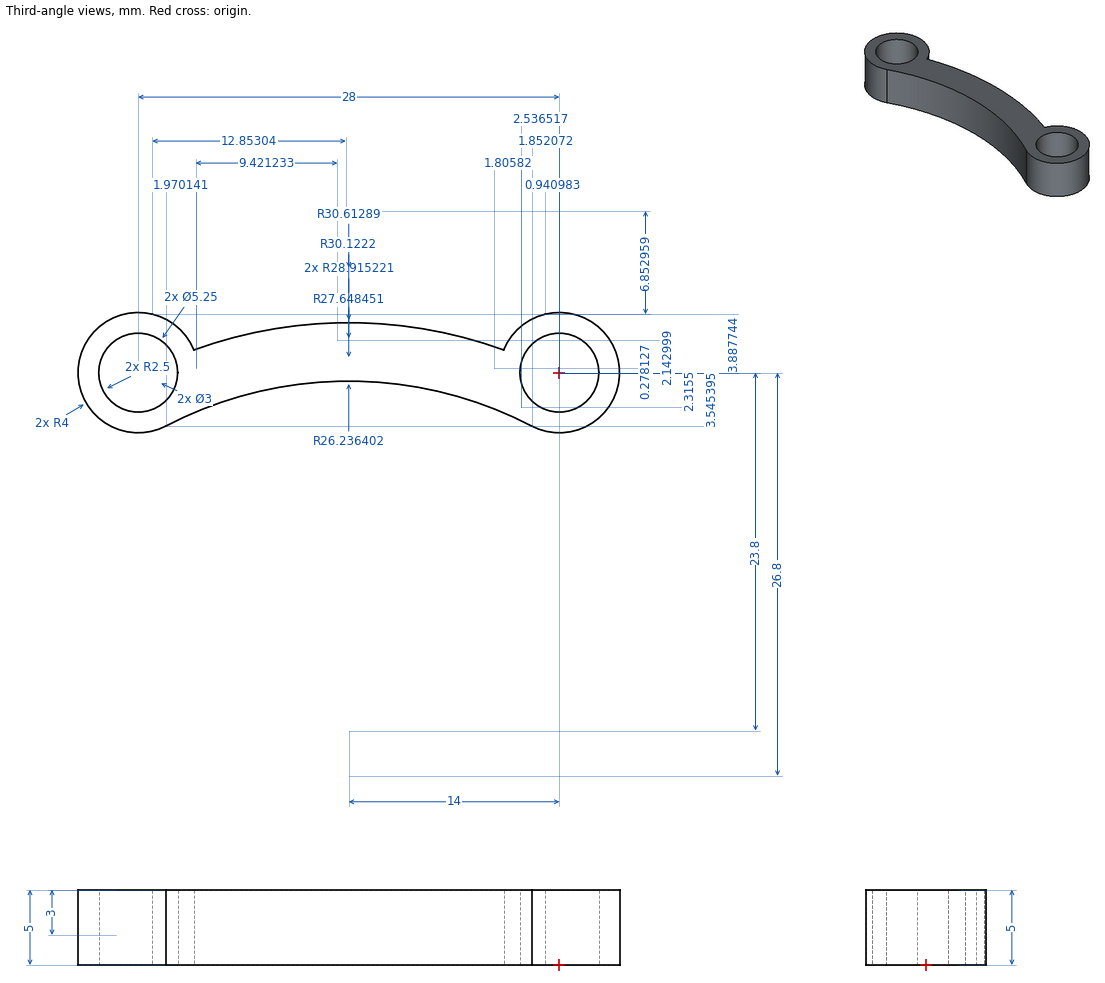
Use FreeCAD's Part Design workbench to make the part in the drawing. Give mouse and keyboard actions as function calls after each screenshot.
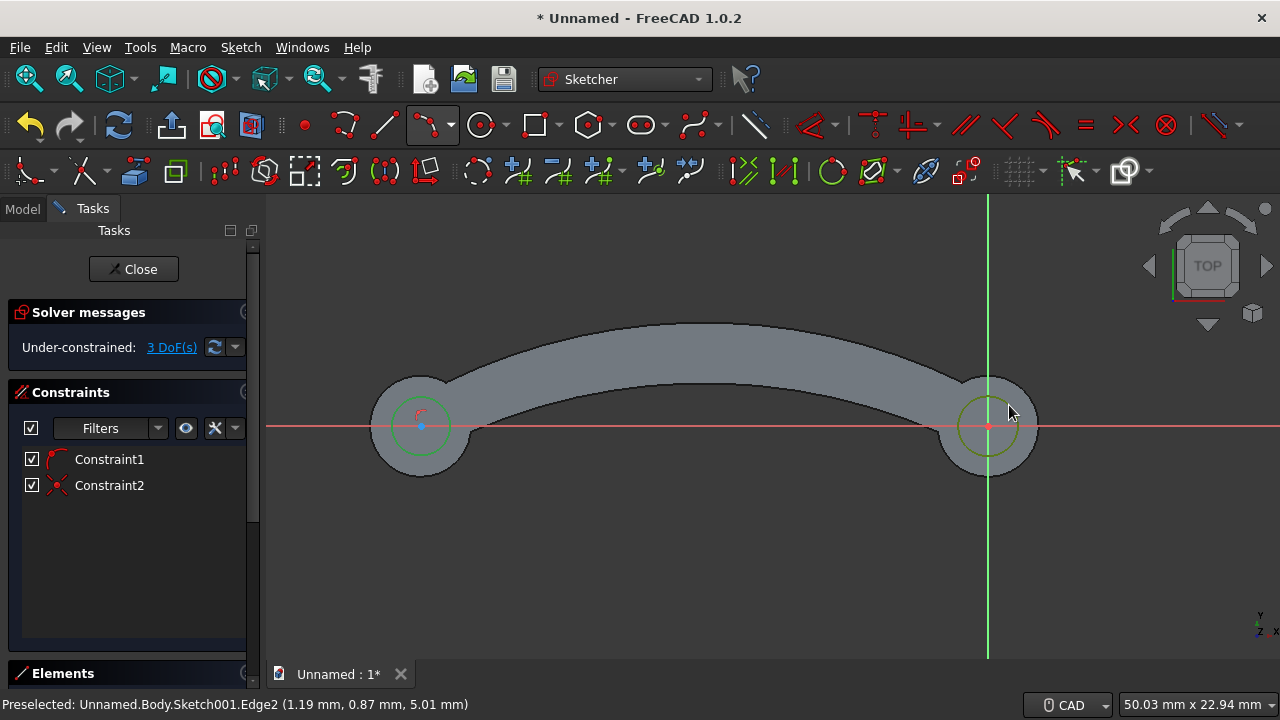
click(1086, 126)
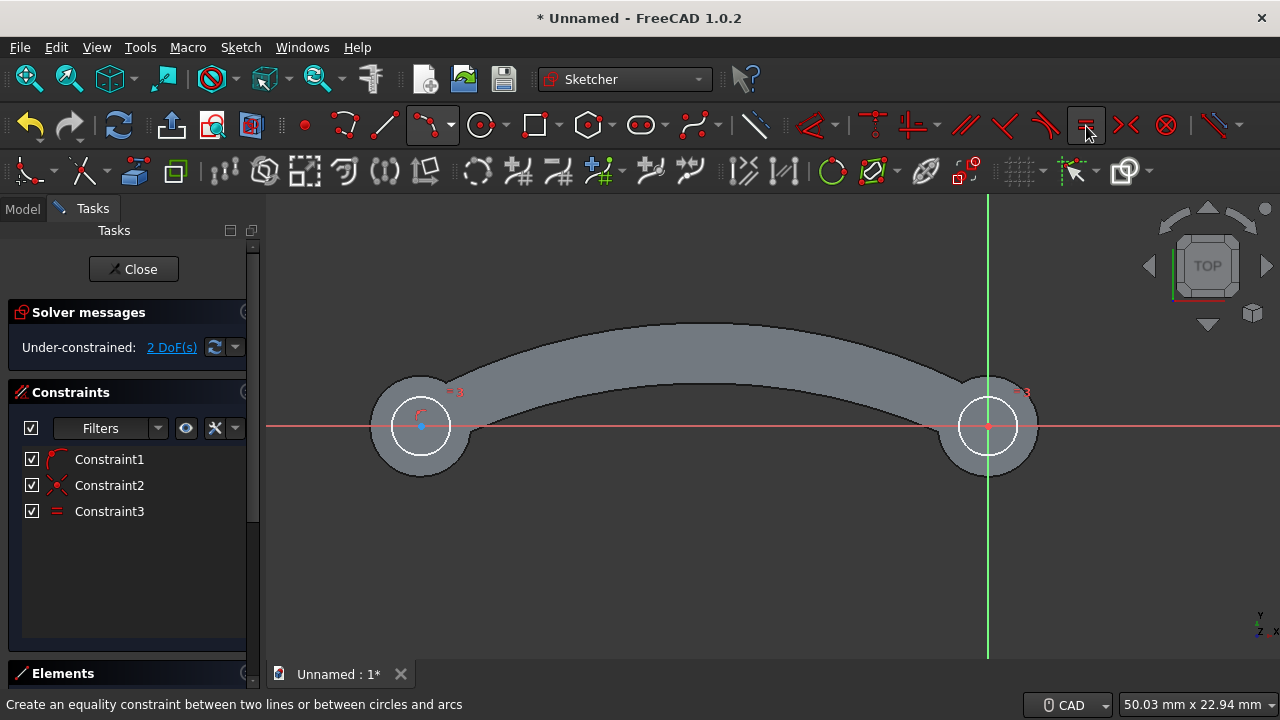
key(d)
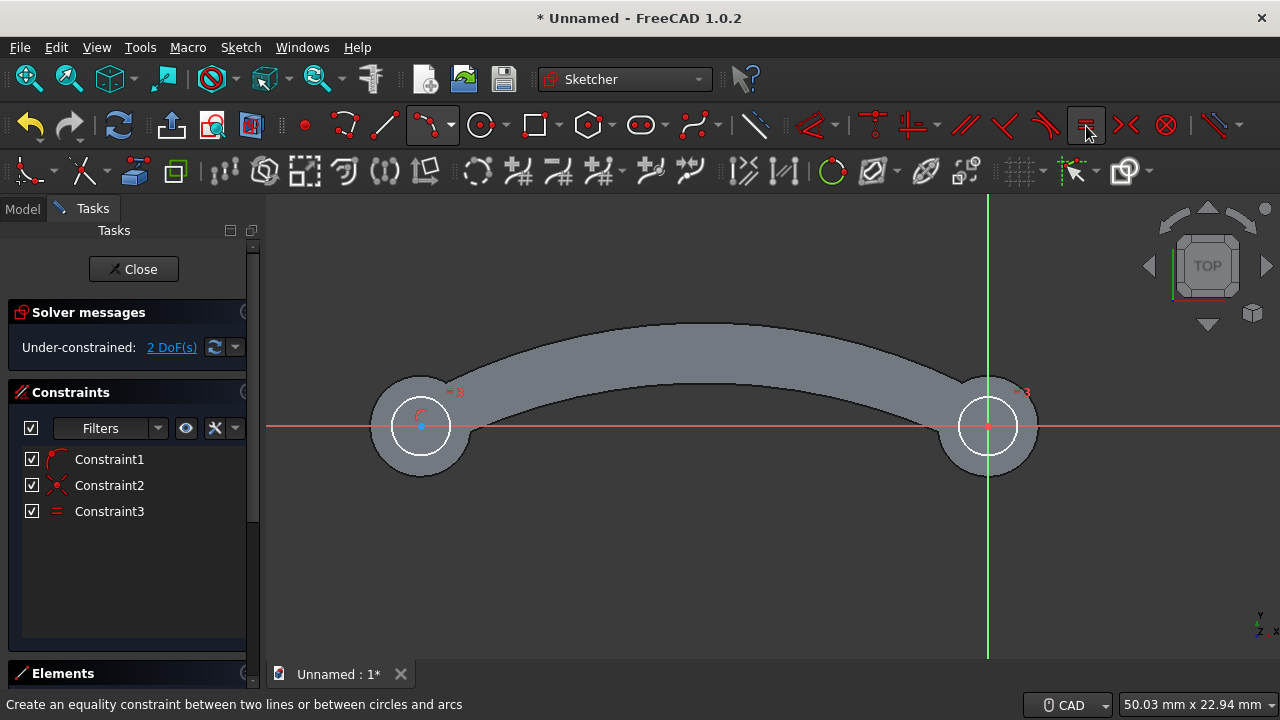
click(442, 406)
click(465, 384)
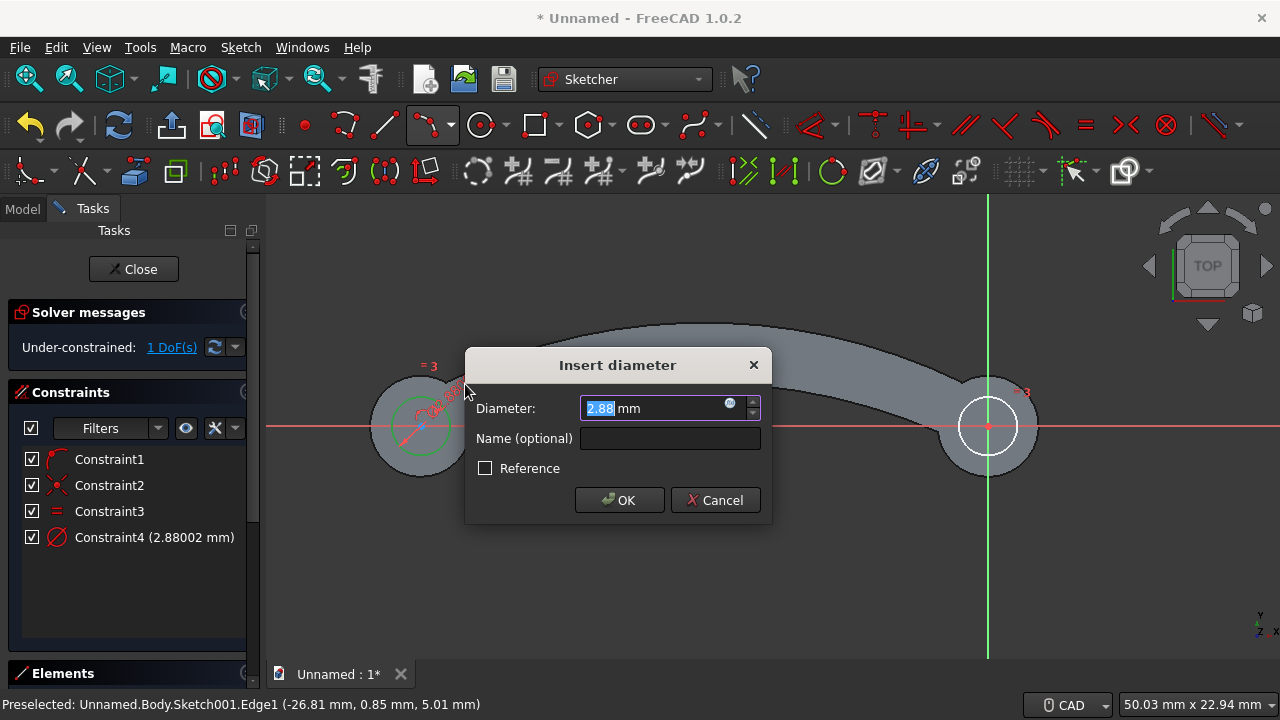
text(3)
key(Return)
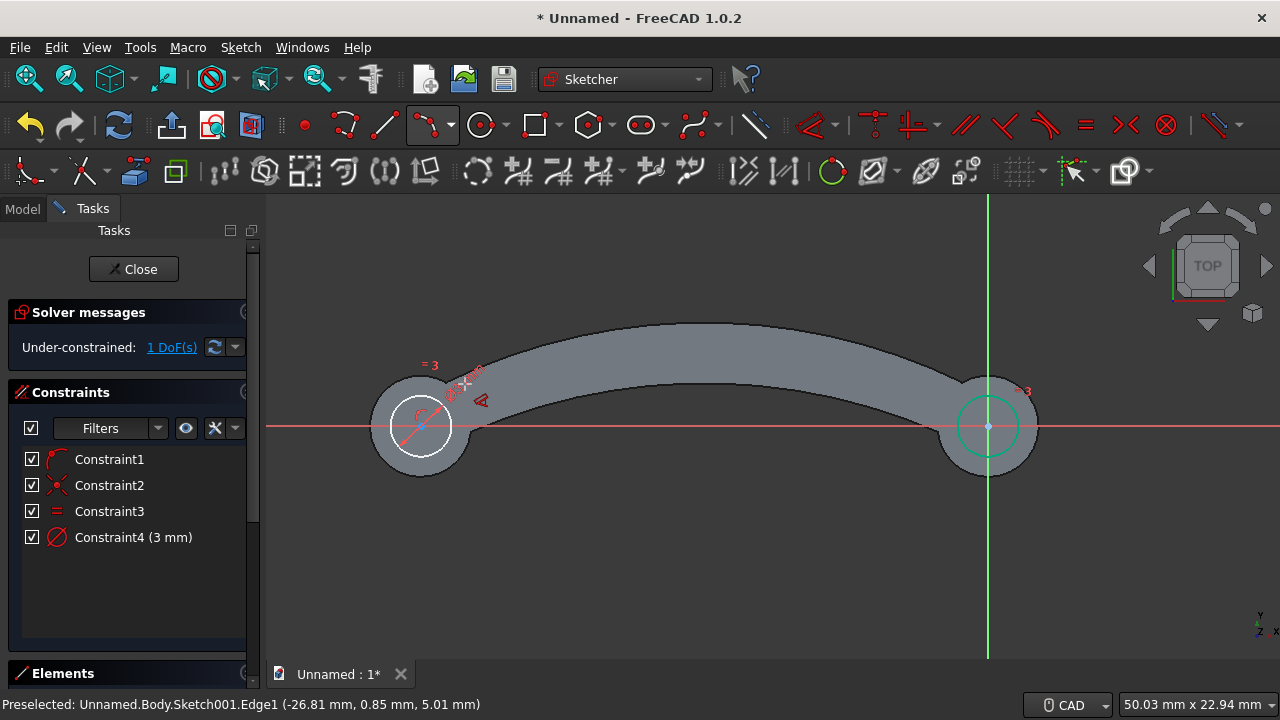
click(421, 426)
click(705, 460)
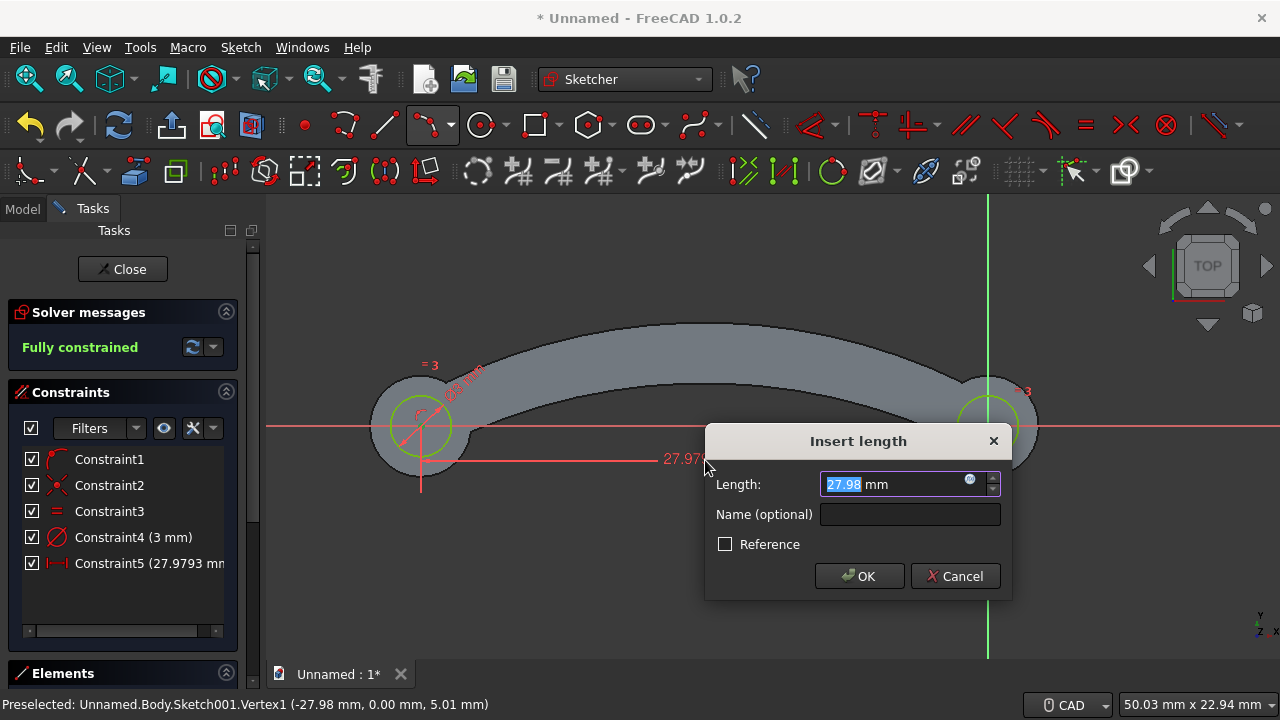
text(28)
key(Return)
key(Escape)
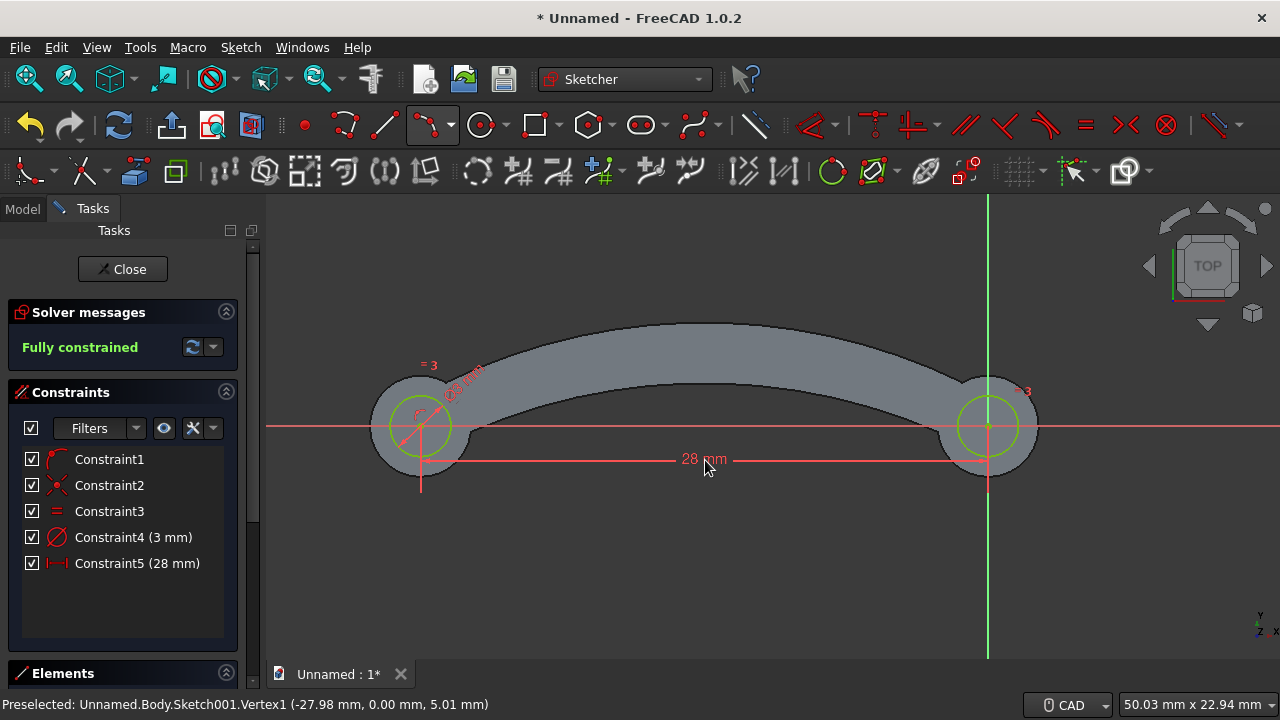
click(123, 269)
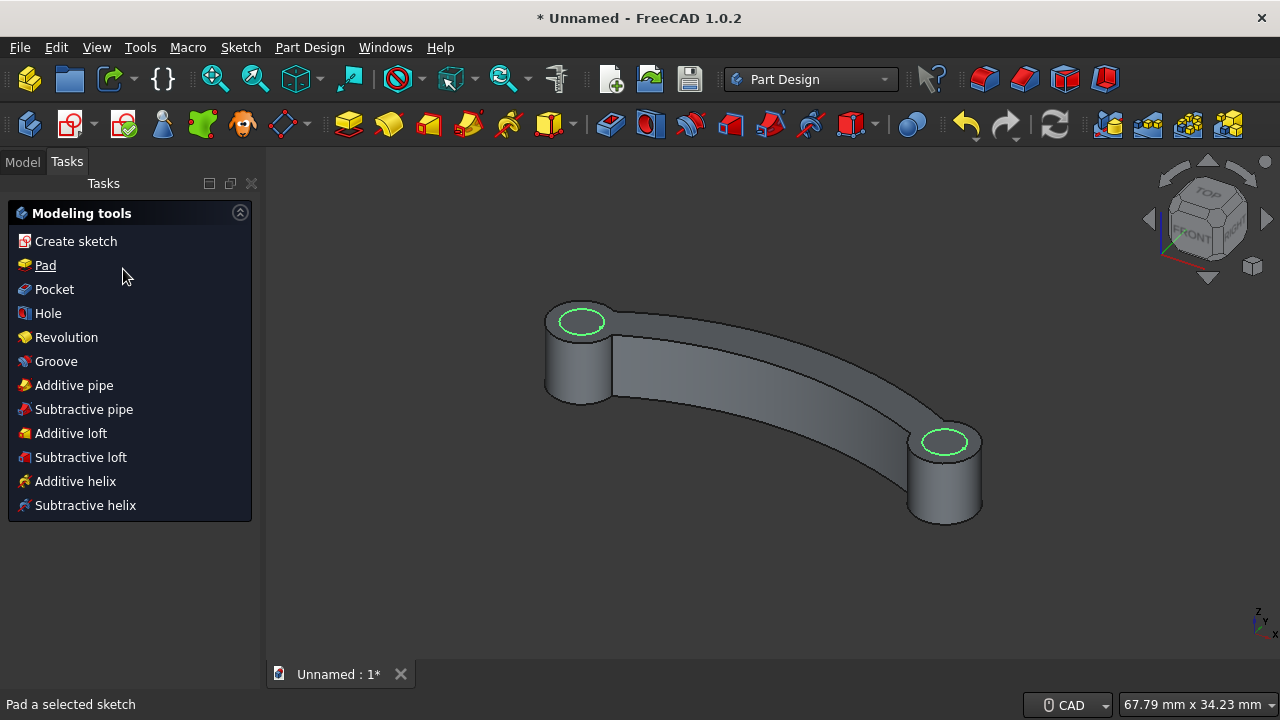
click(612, 124)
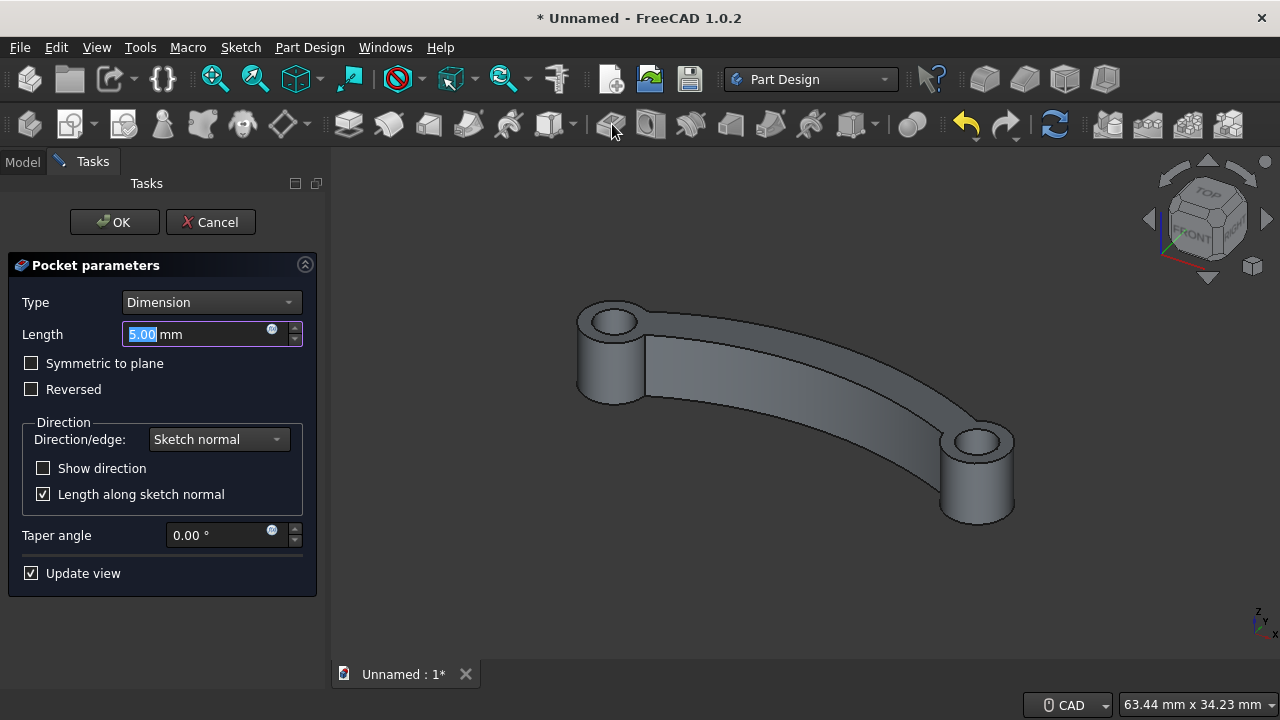
text(3)
key(Tab)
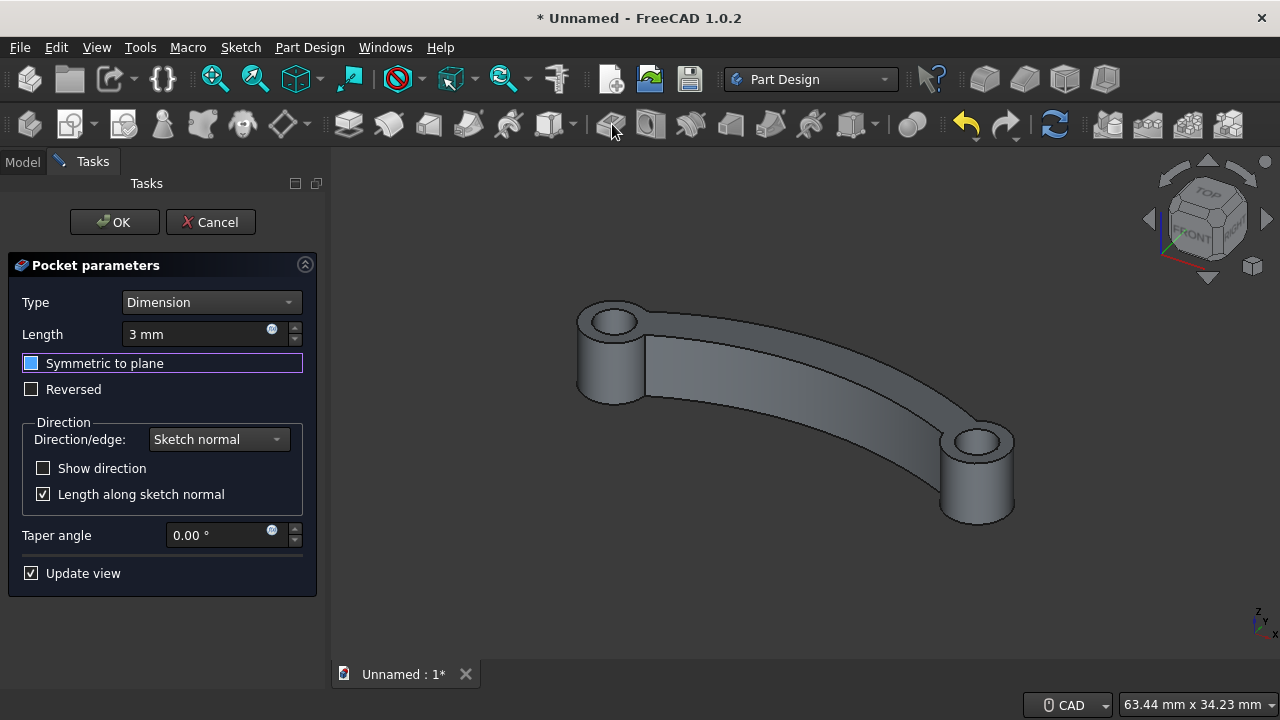
click(115, 222)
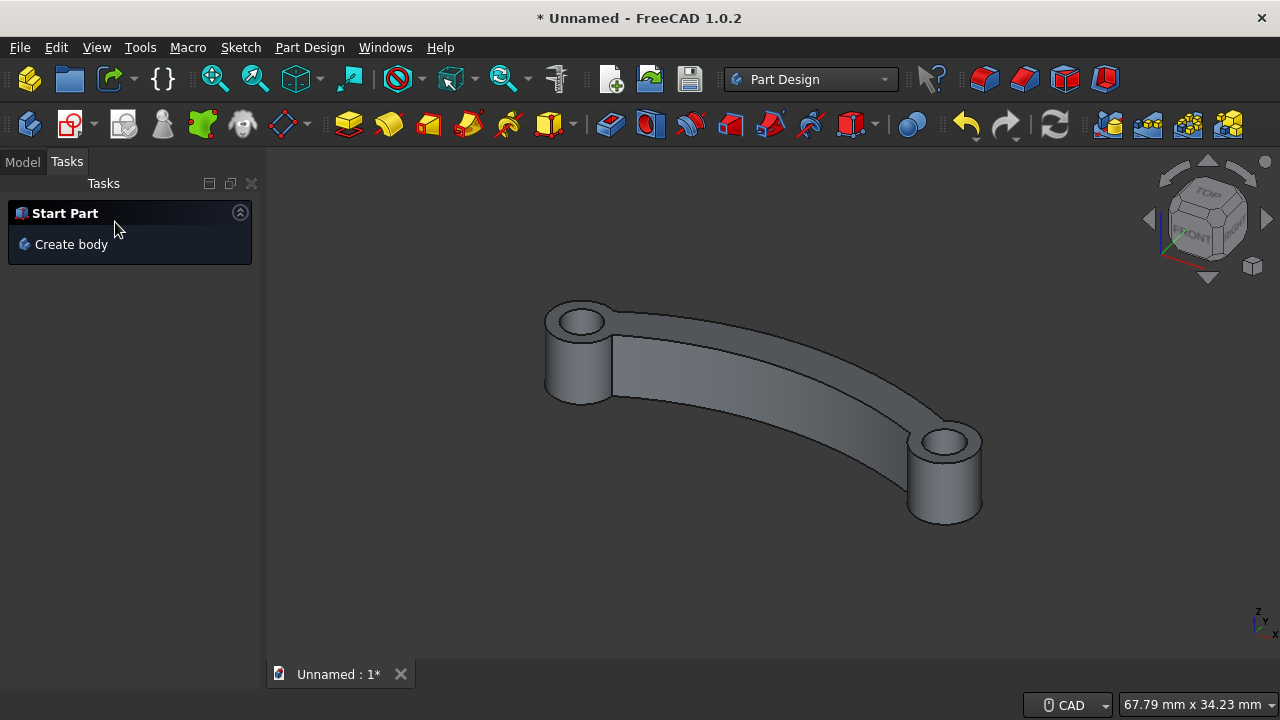
click(789, 355)